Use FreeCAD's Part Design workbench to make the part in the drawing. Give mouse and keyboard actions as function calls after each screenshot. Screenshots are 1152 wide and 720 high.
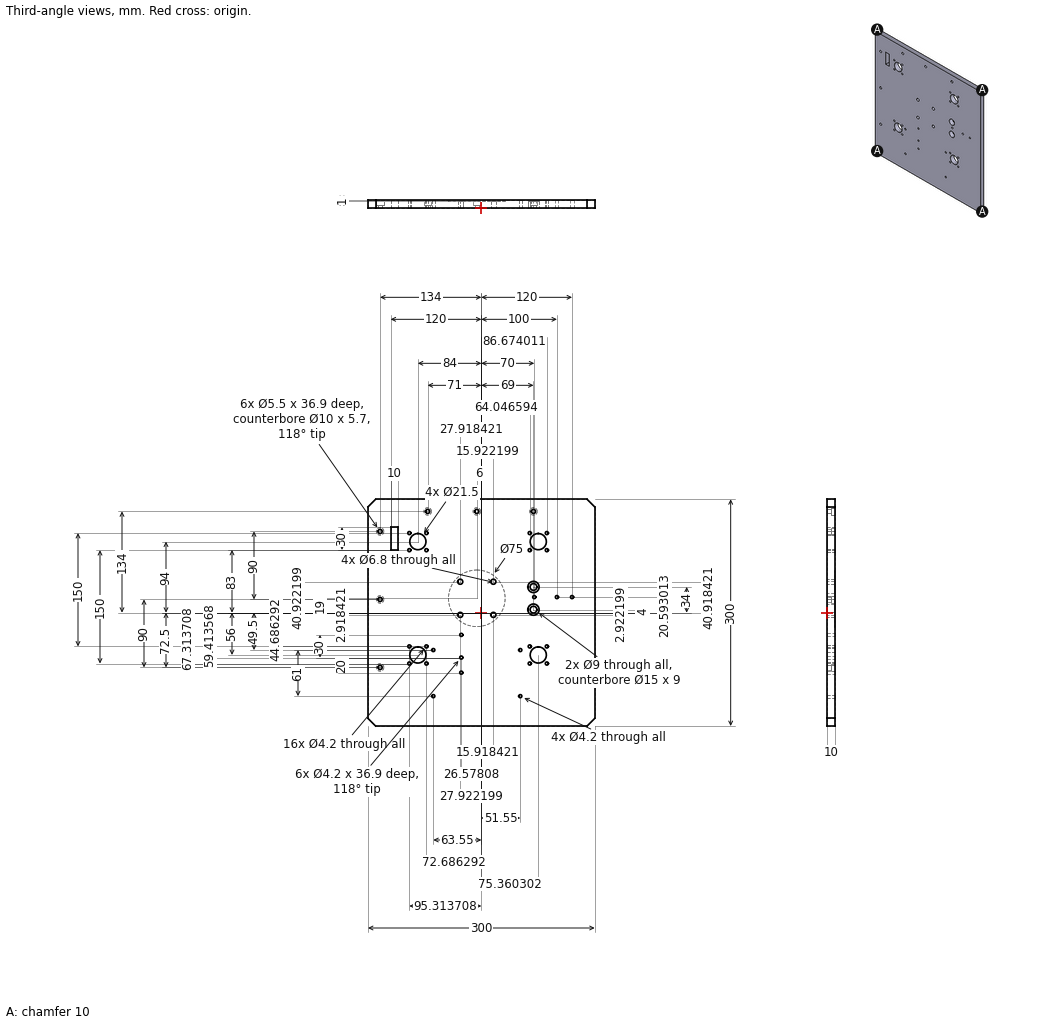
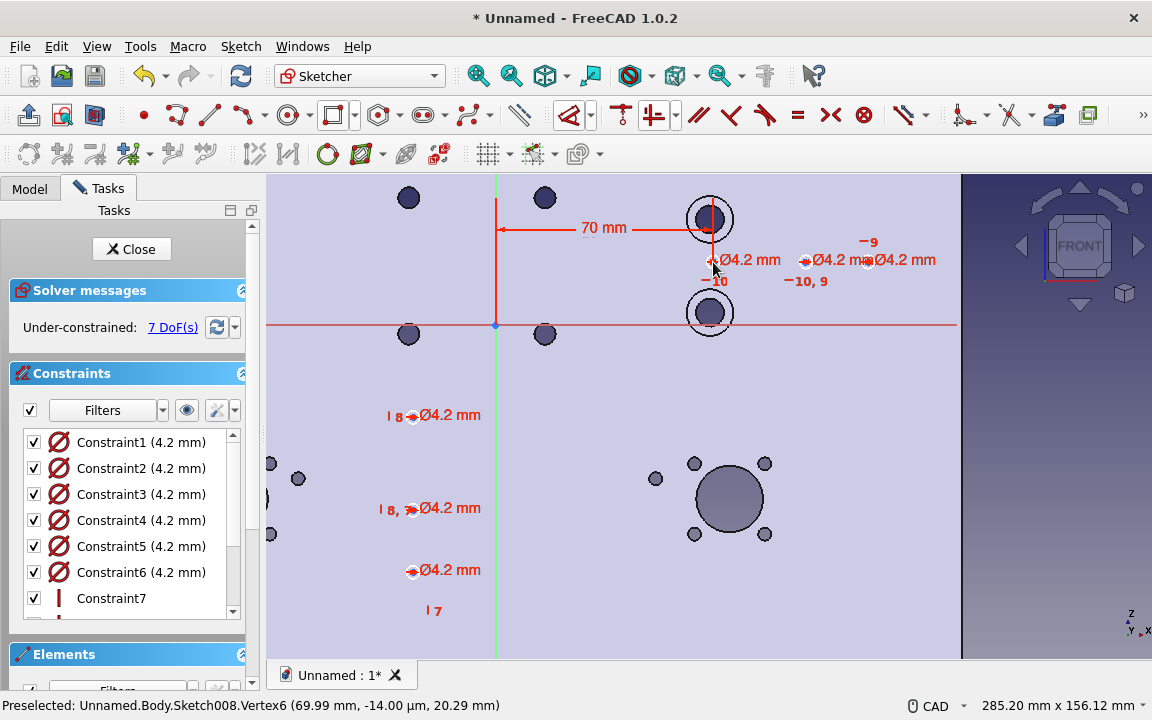
click(806, 262)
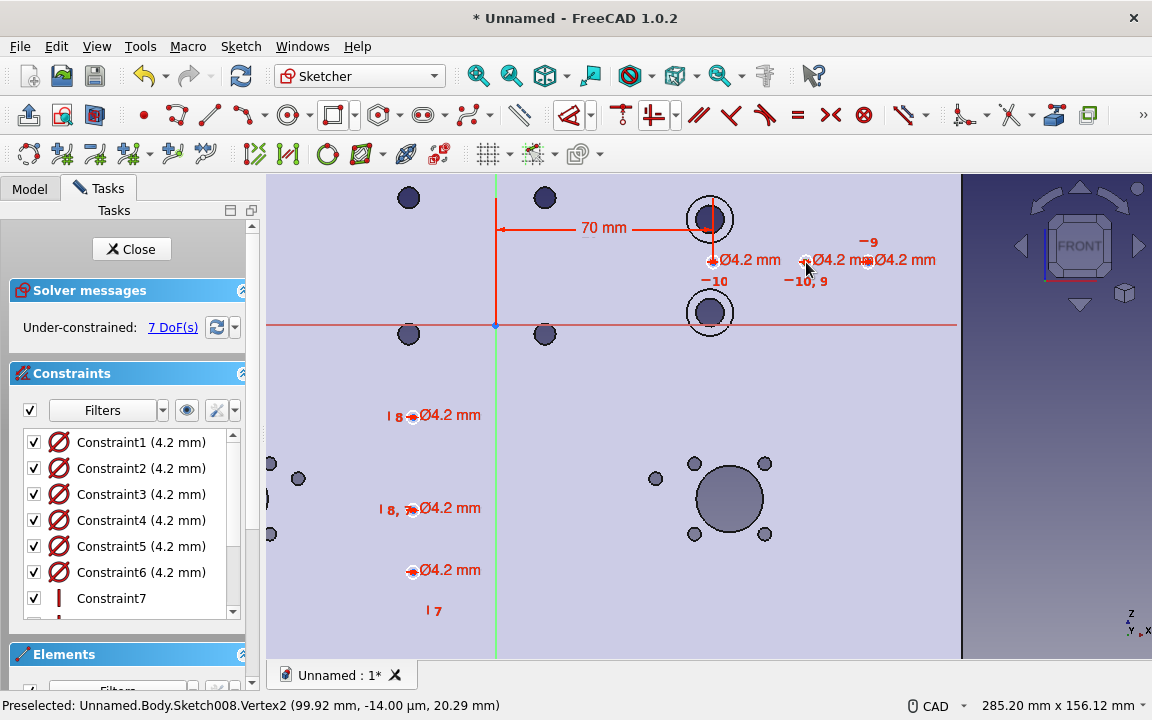
click(590, 116)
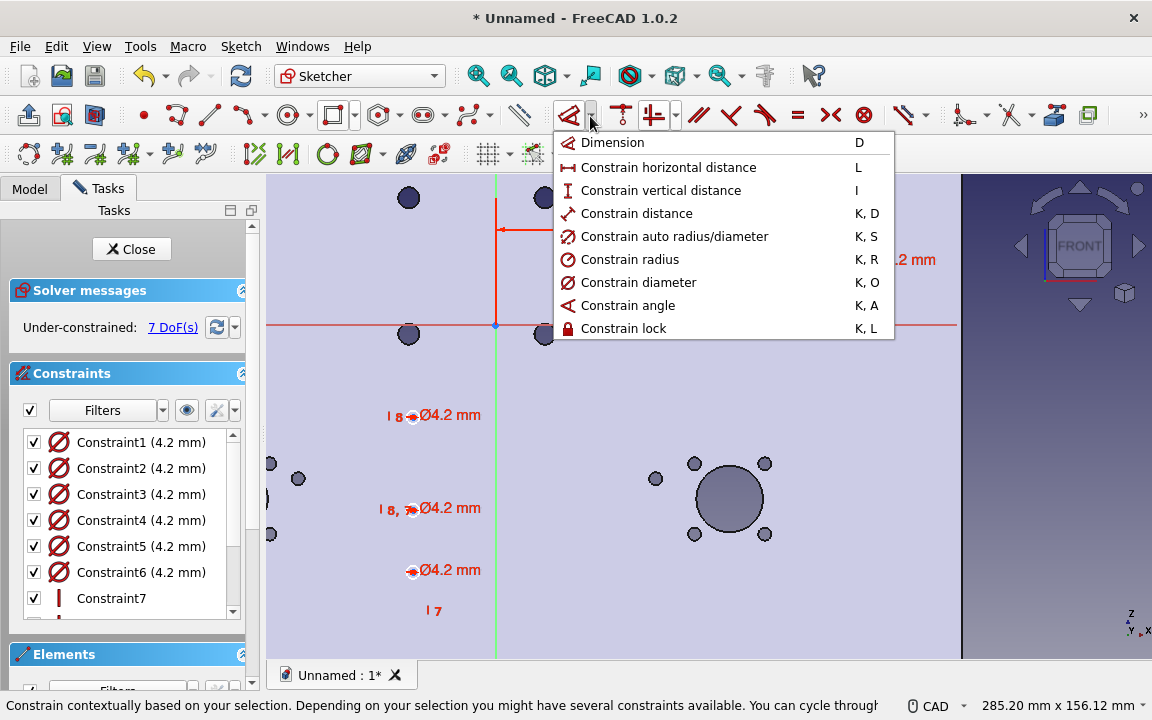
click(724, 168)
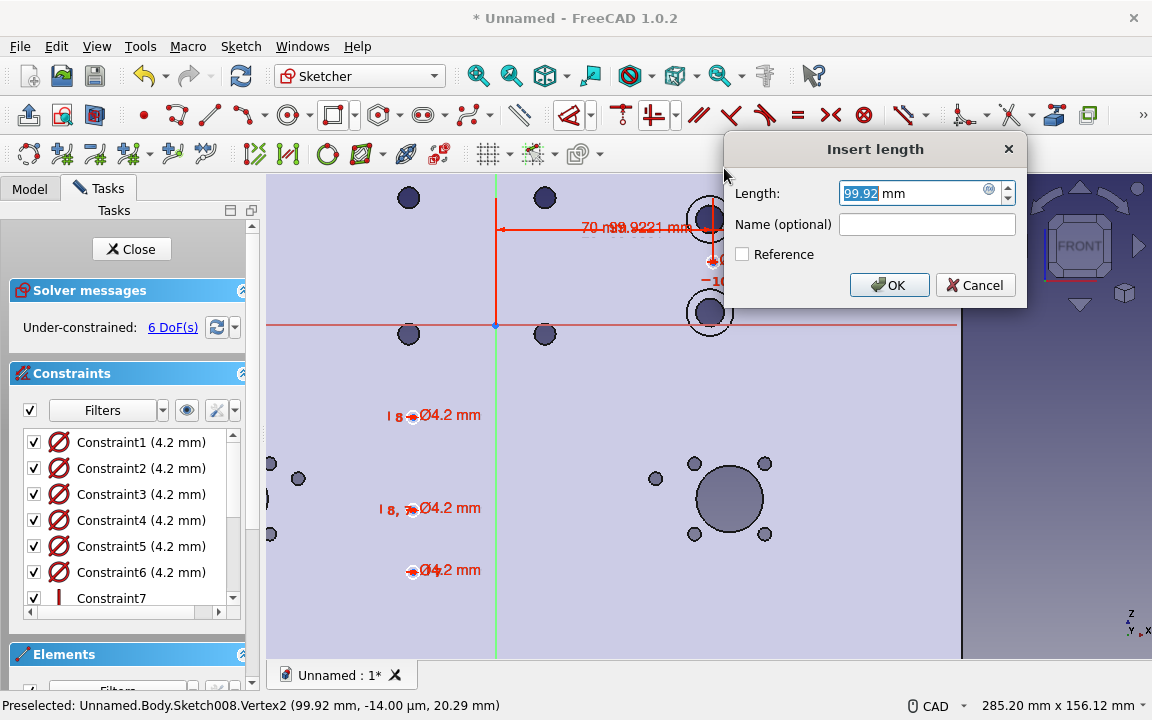
text(100)
key(Return)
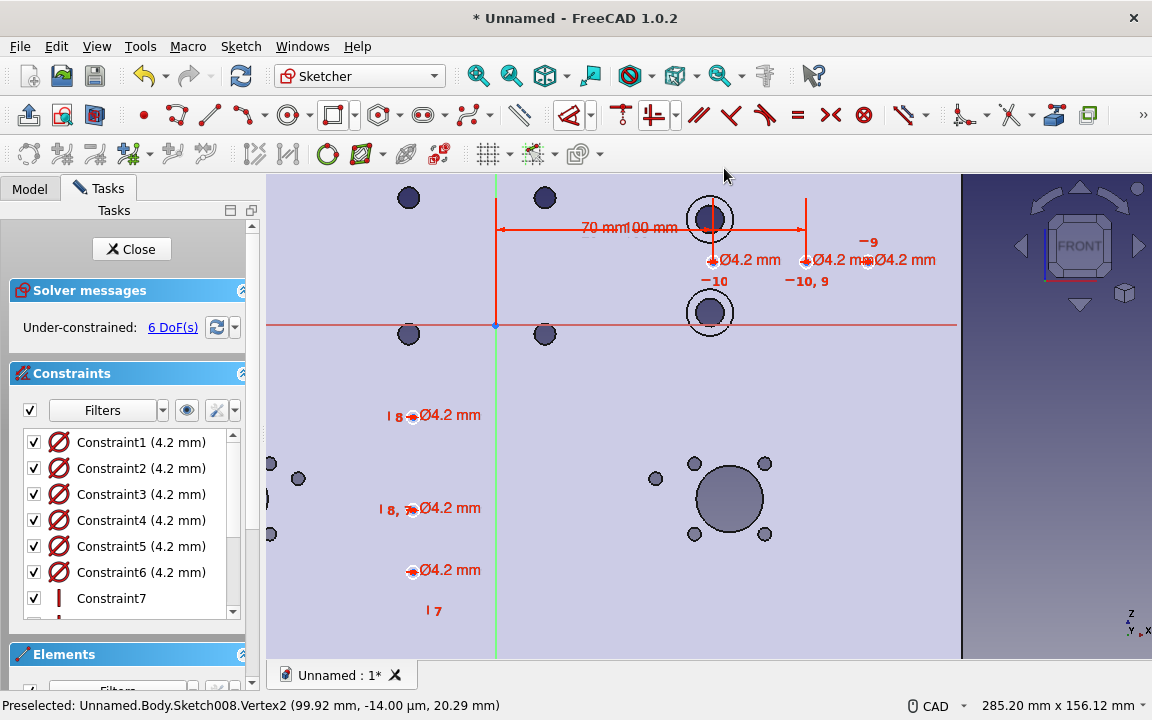
click(868, 262)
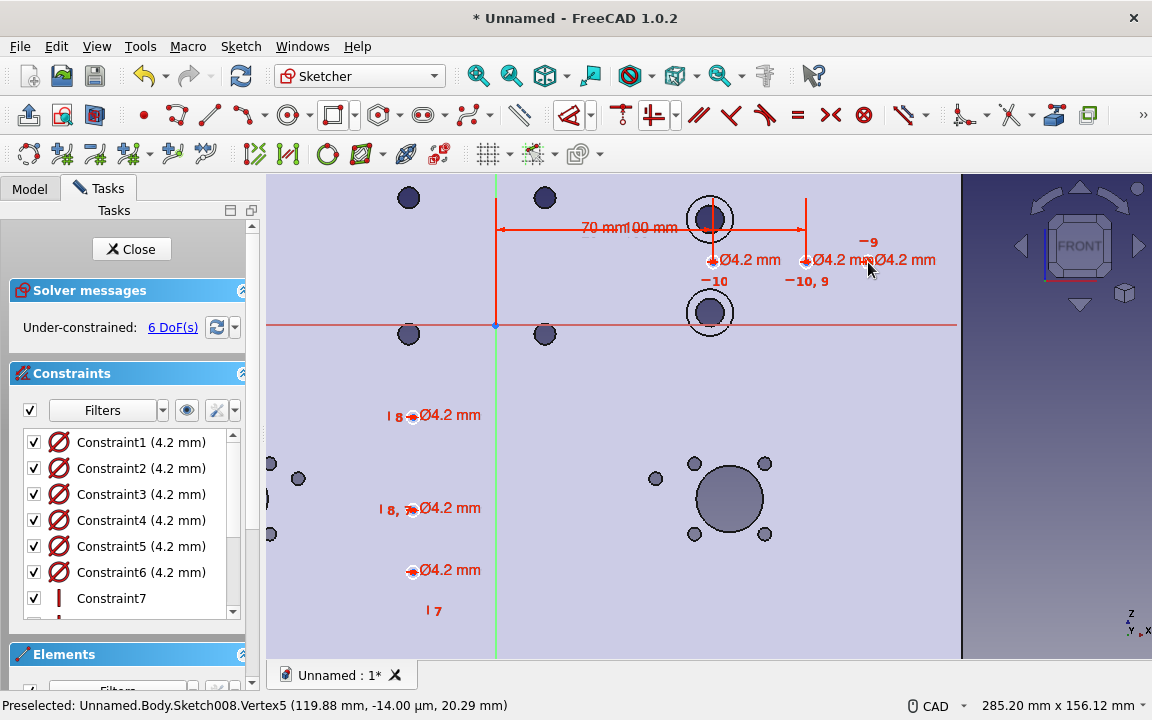
key(l)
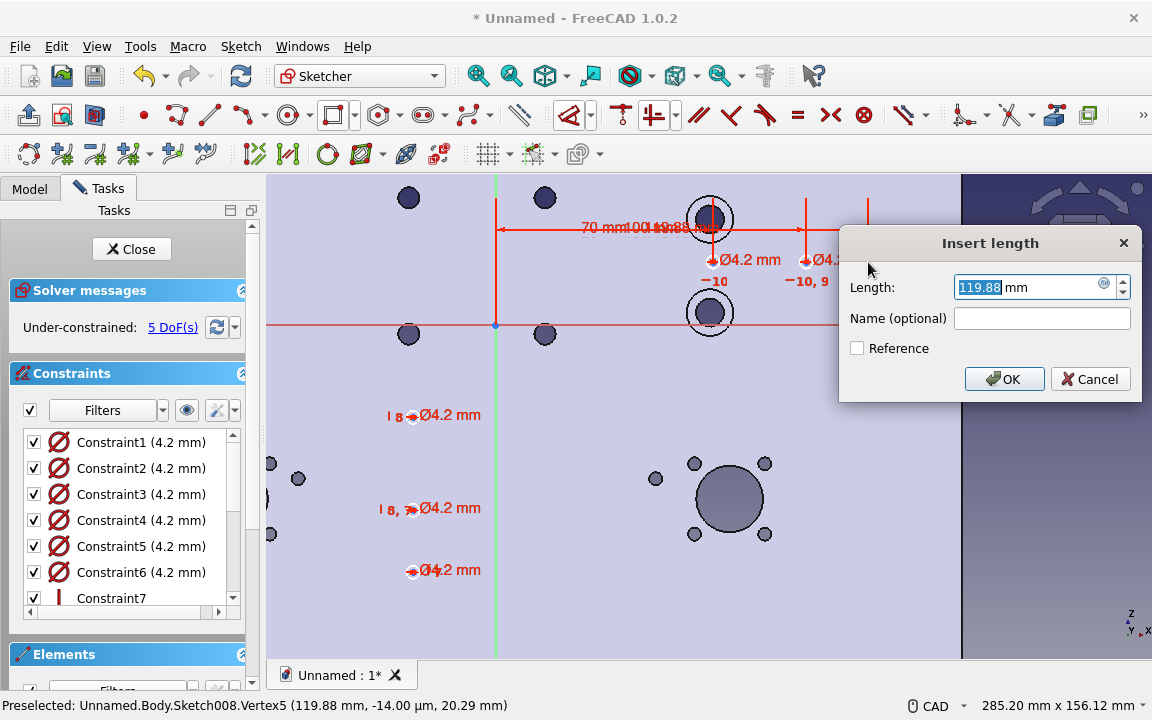
text(120)
key(Return)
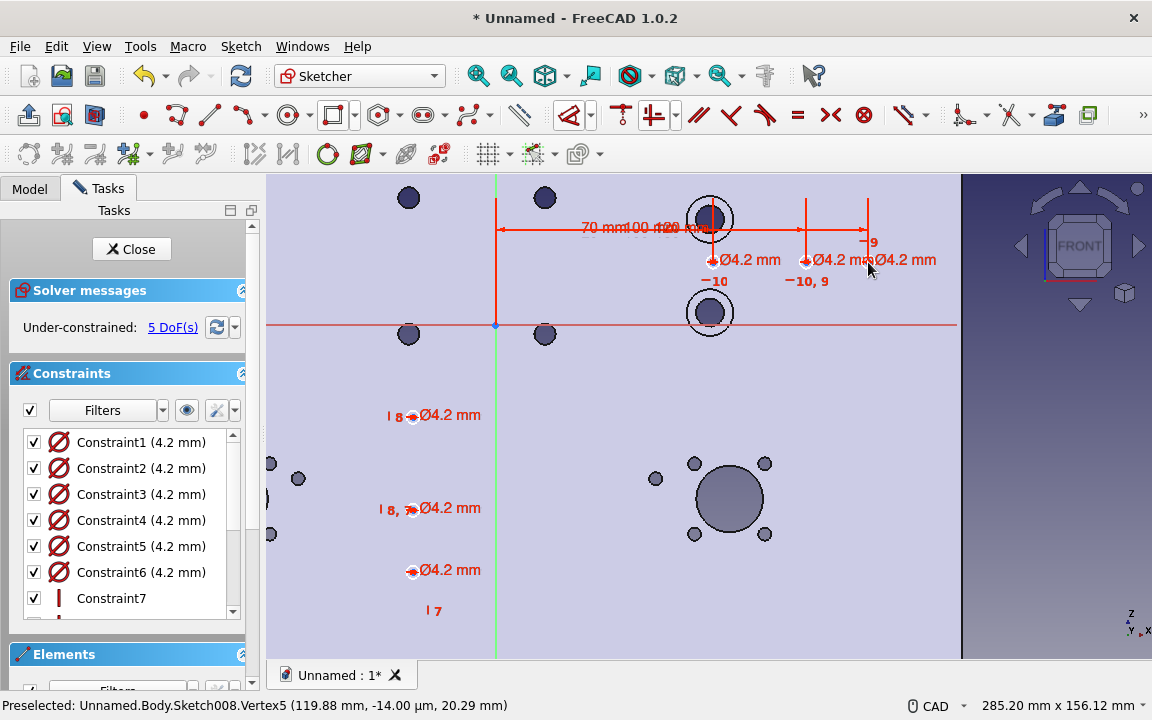
click(413, 510)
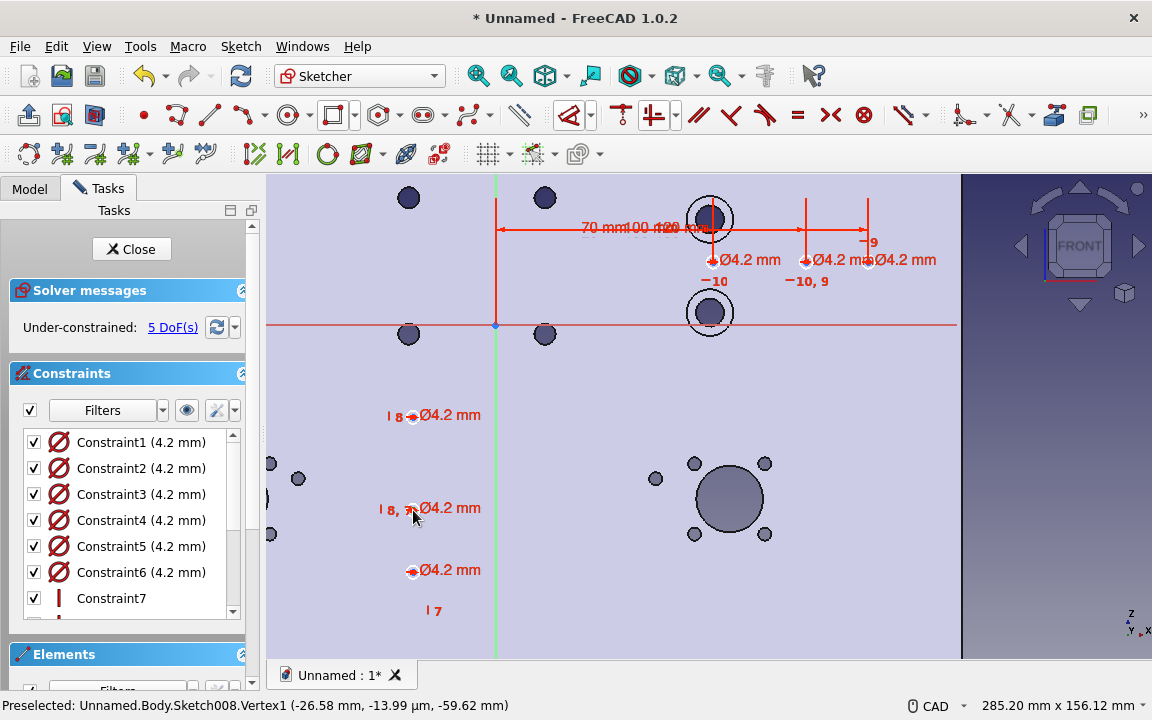
click(413, 572)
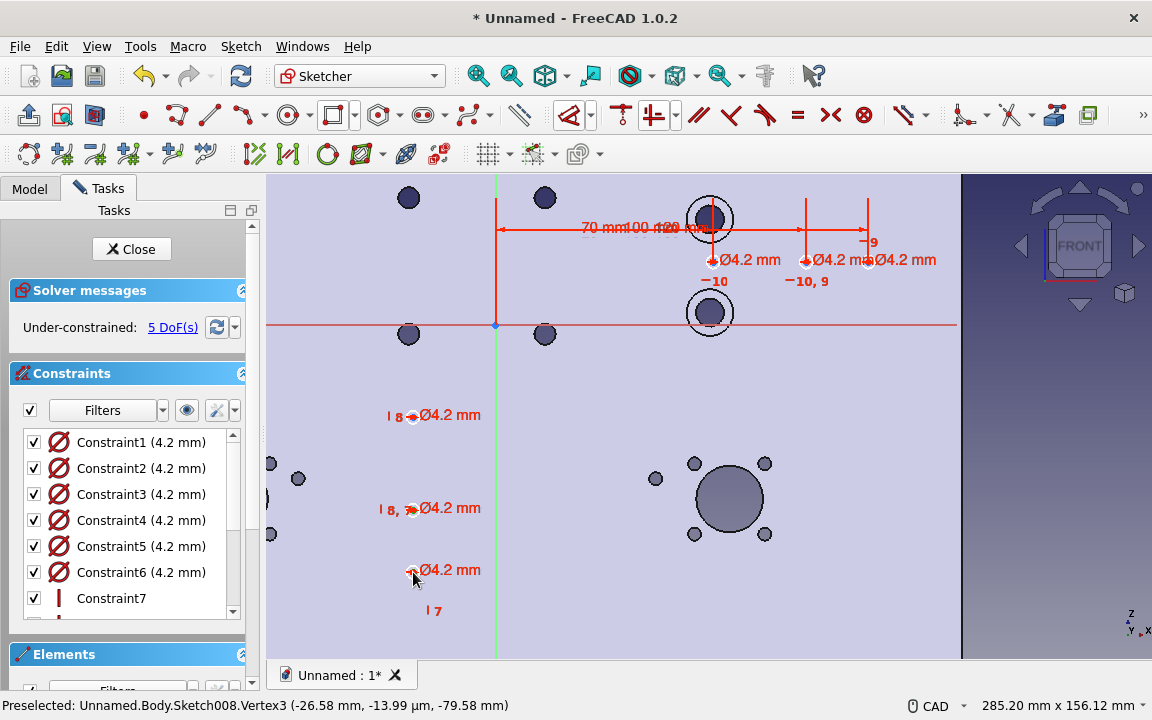
key(i)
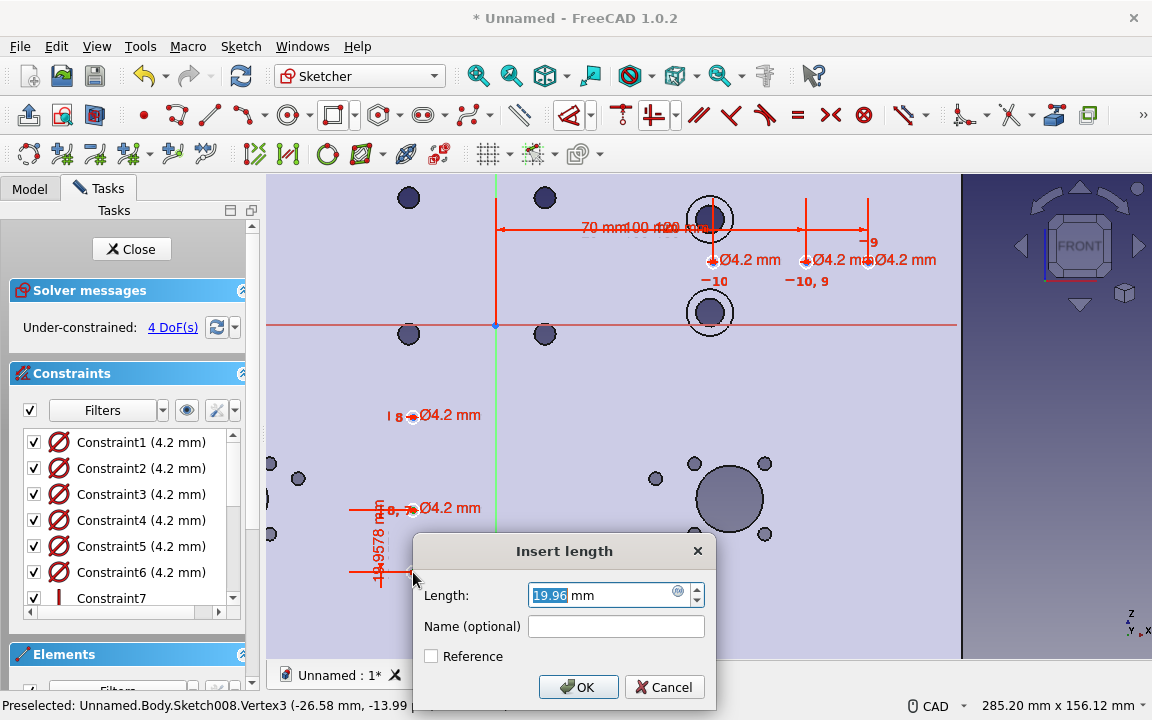
text(20)
key(Return)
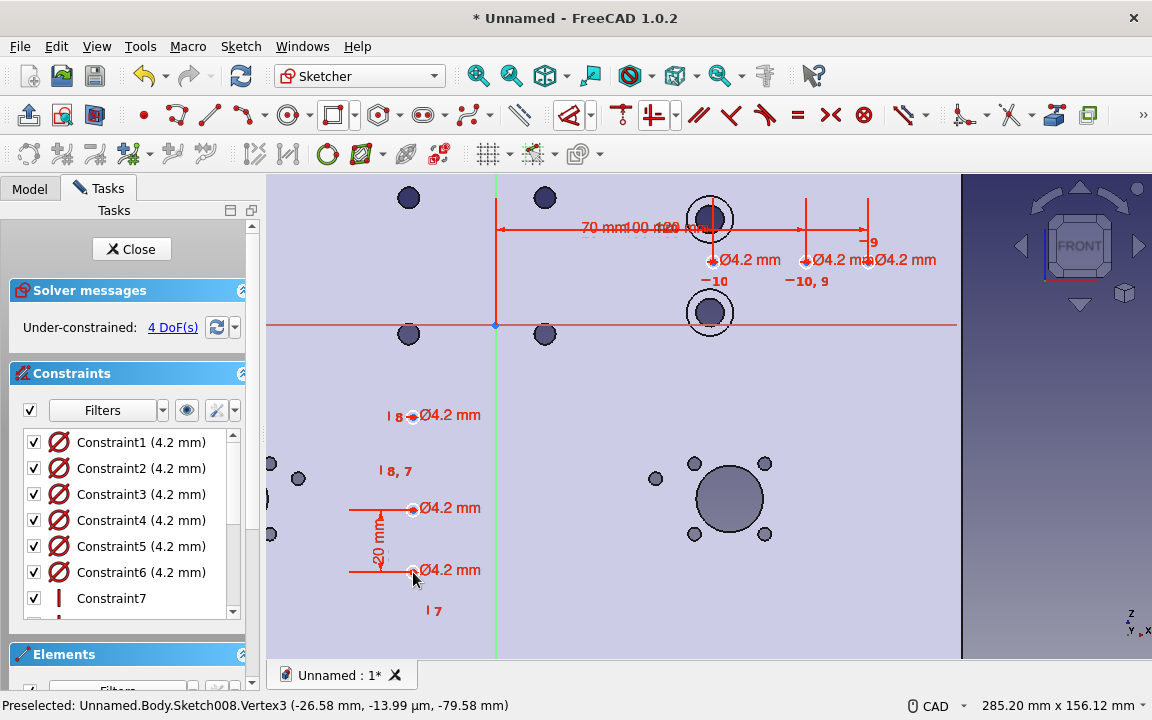
click(413, 510)